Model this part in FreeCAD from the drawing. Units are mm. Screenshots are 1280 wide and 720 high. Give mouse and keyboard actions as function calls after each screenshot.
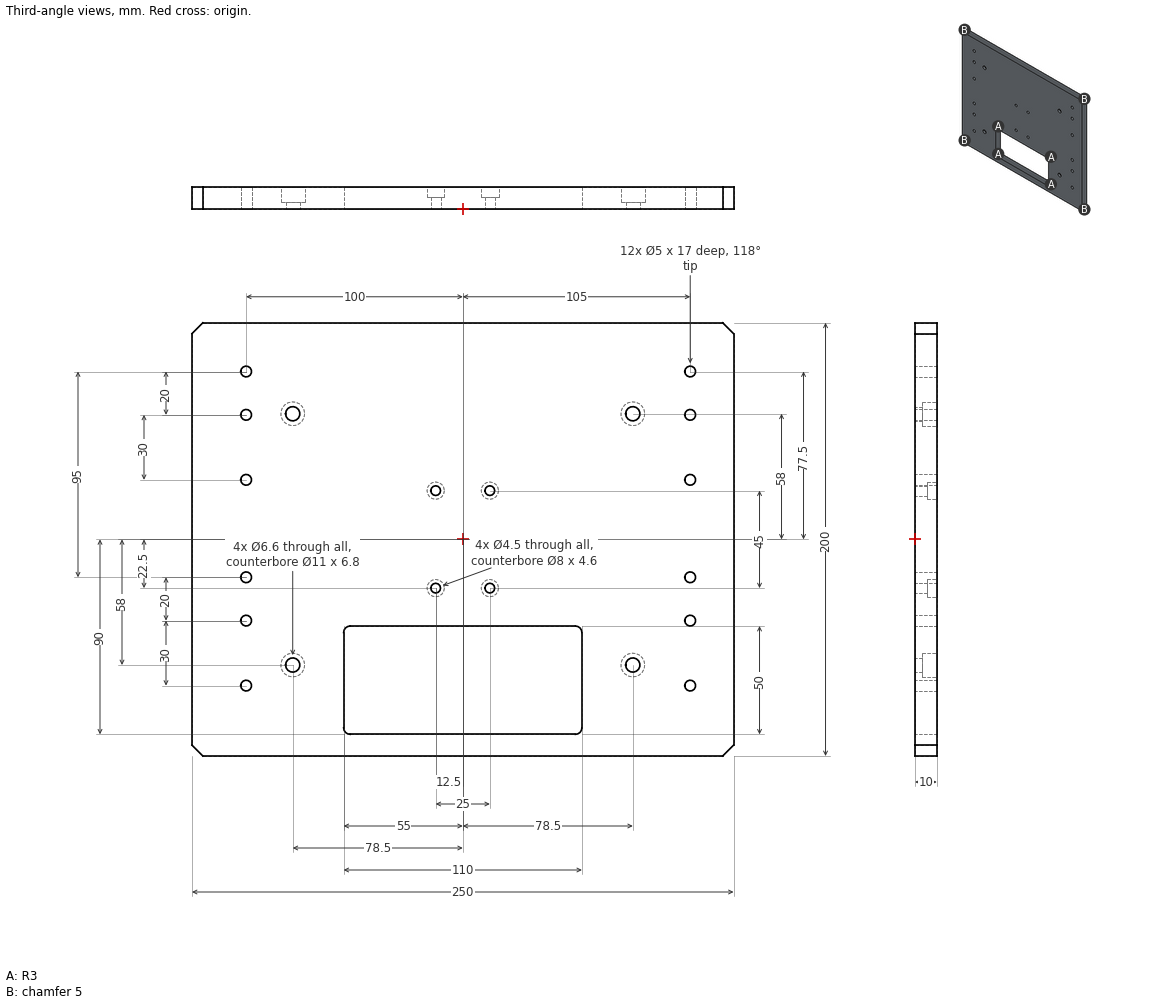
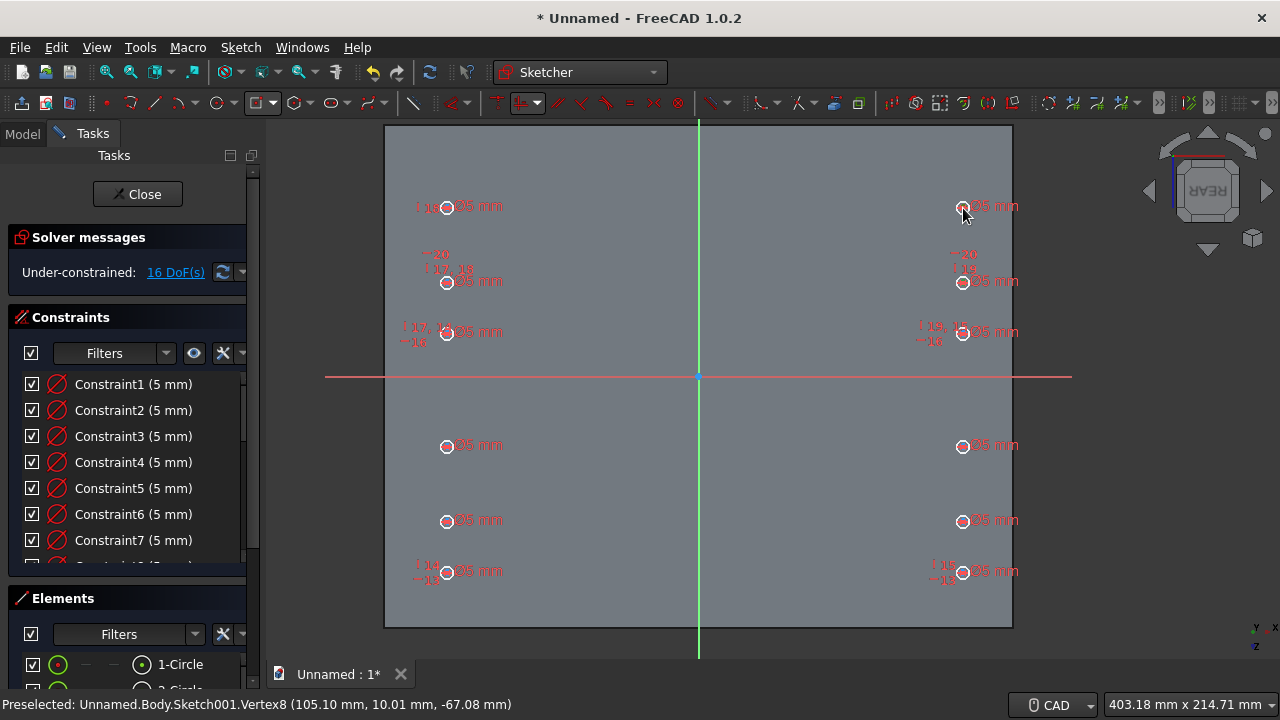
click(540, 104)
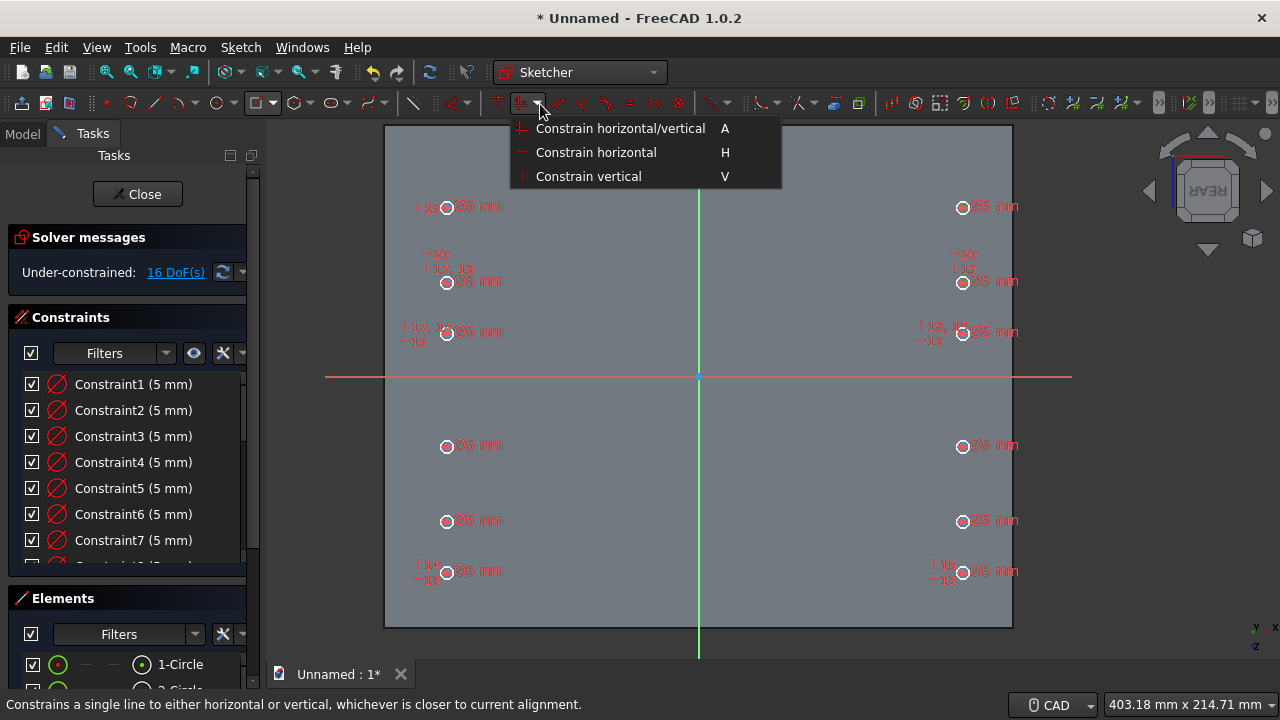
click(646, 176)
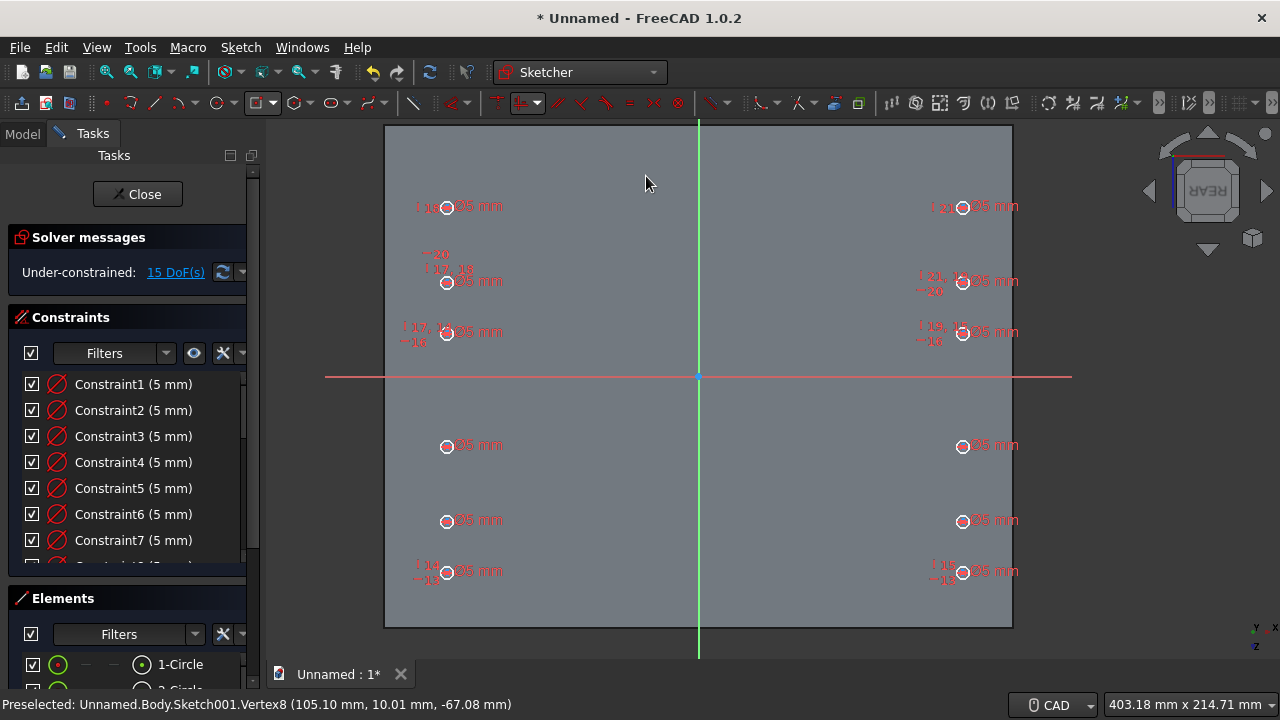
click(447, 208)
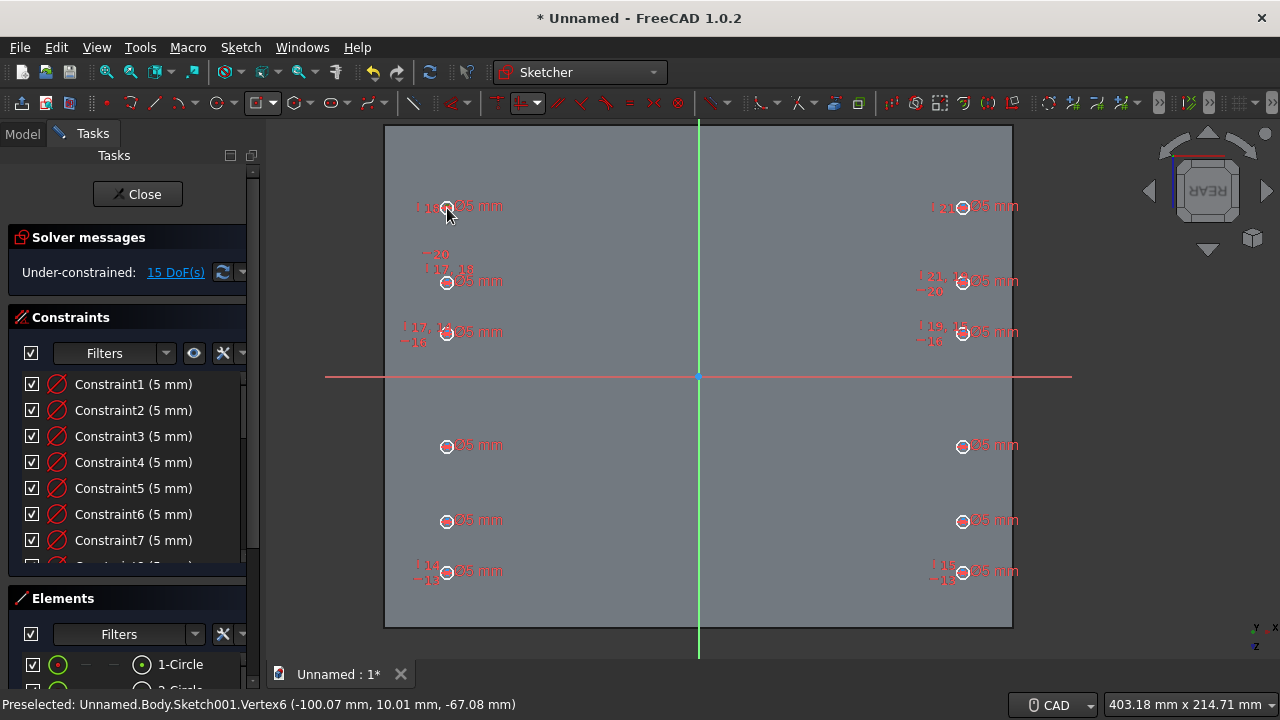
click(963, 208)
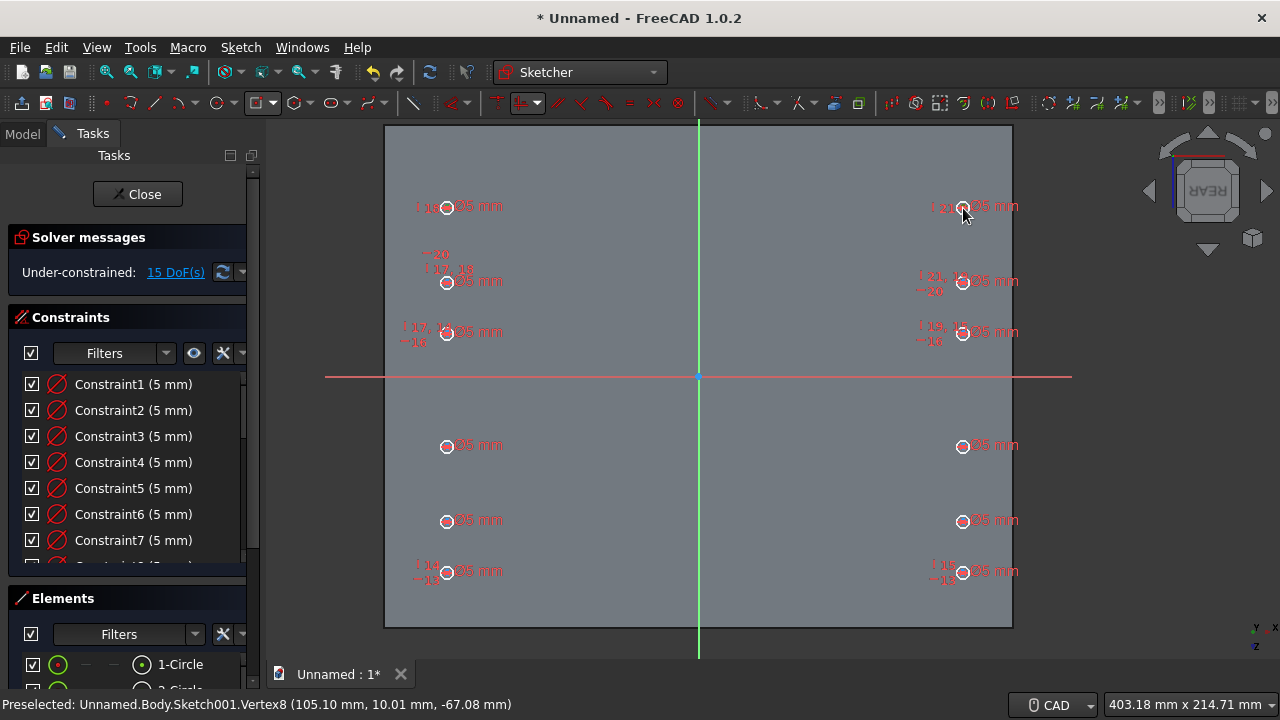
key(h)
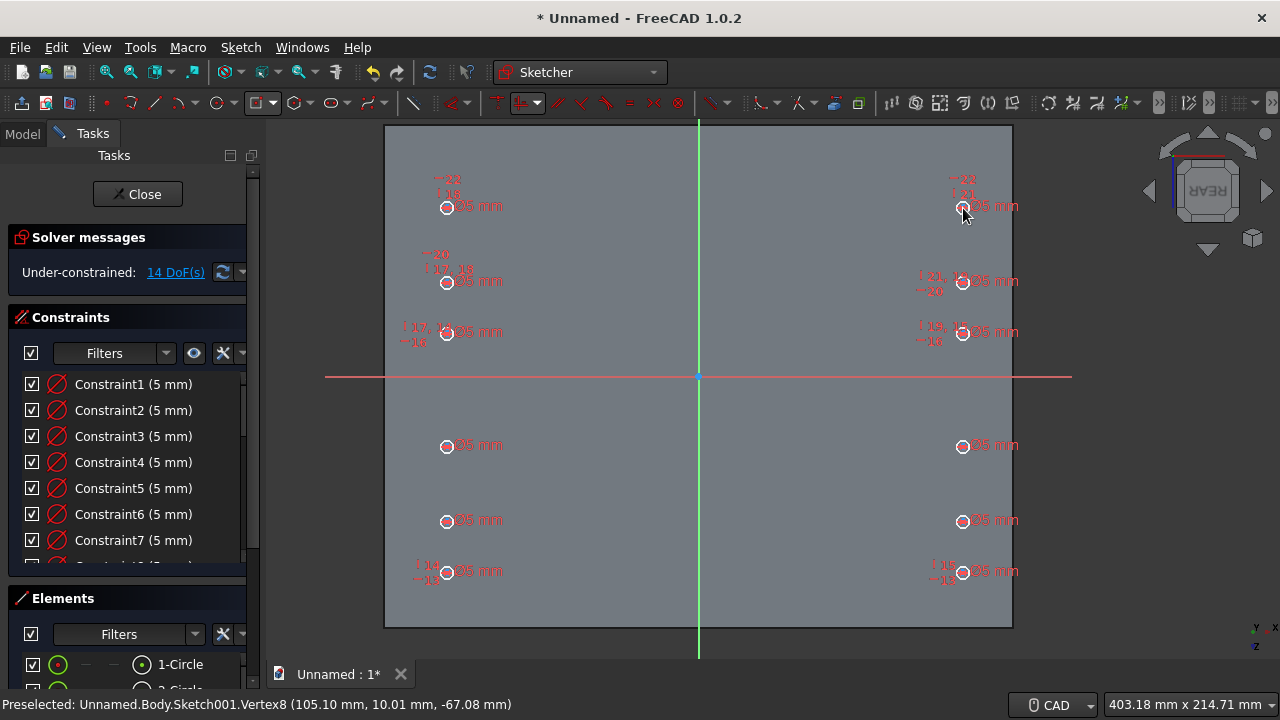
click(447, 573)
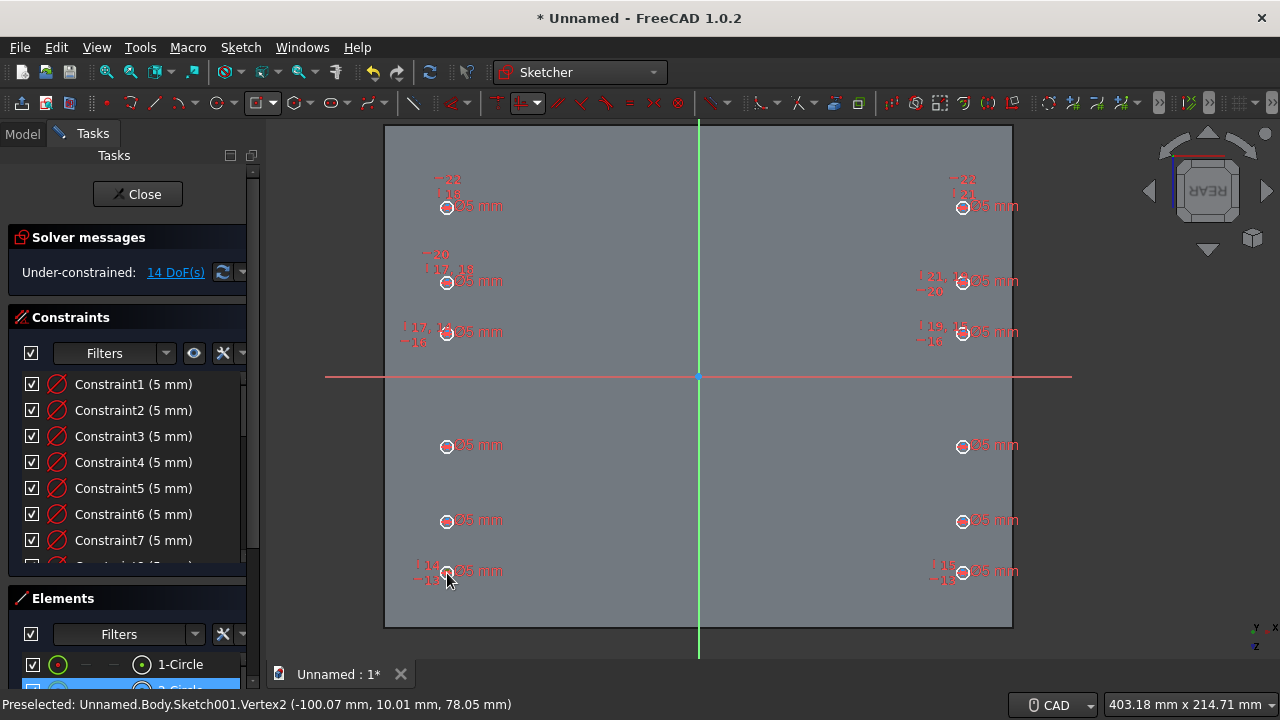
click(447, 522)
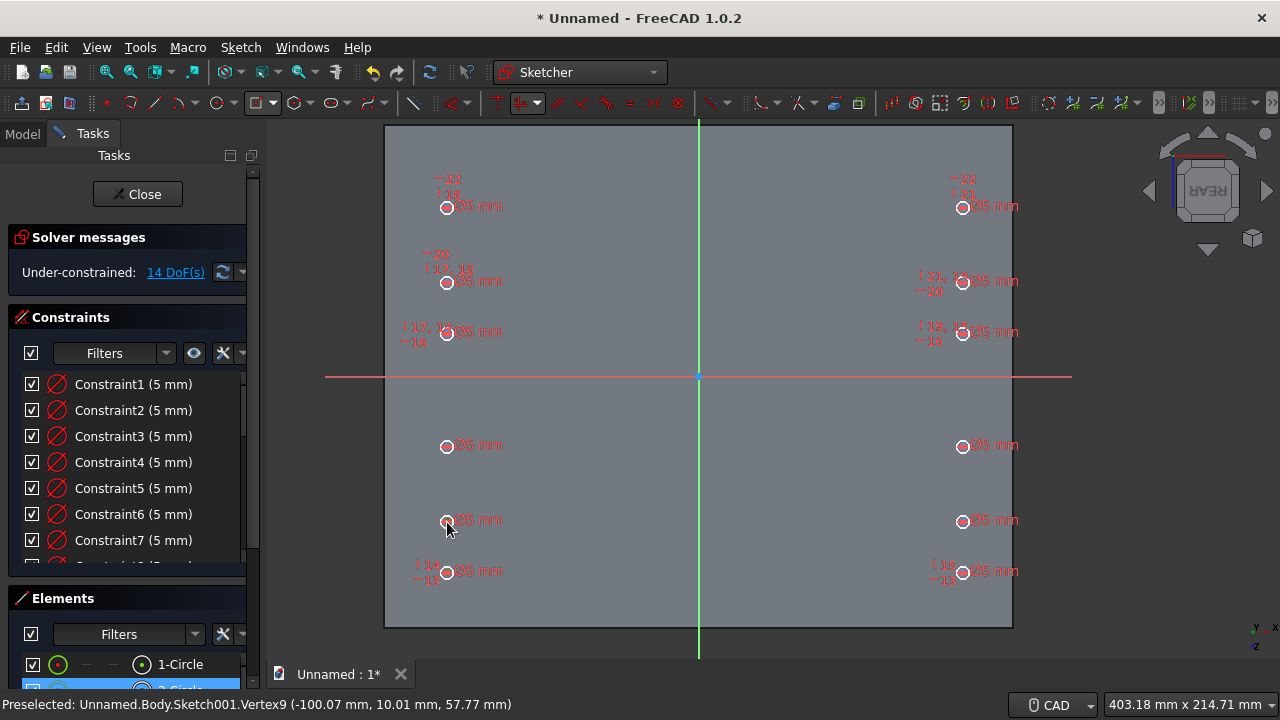
click(540, 104)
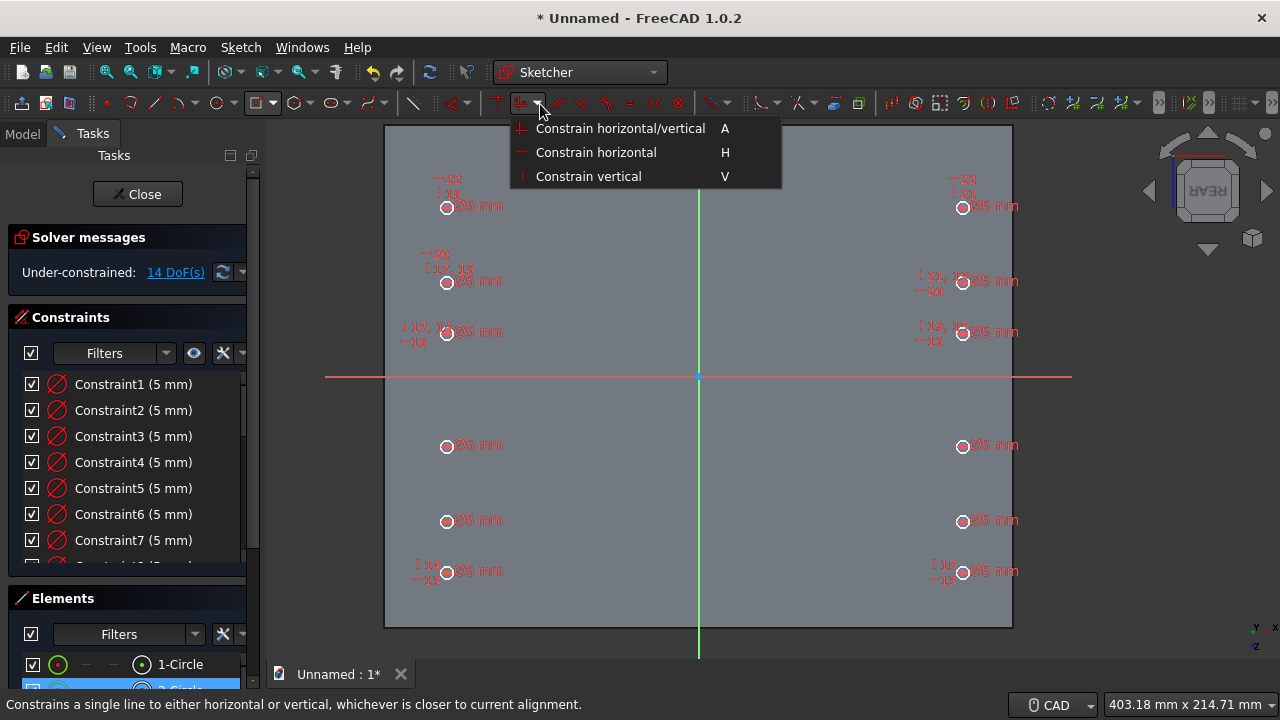
click(646, 176)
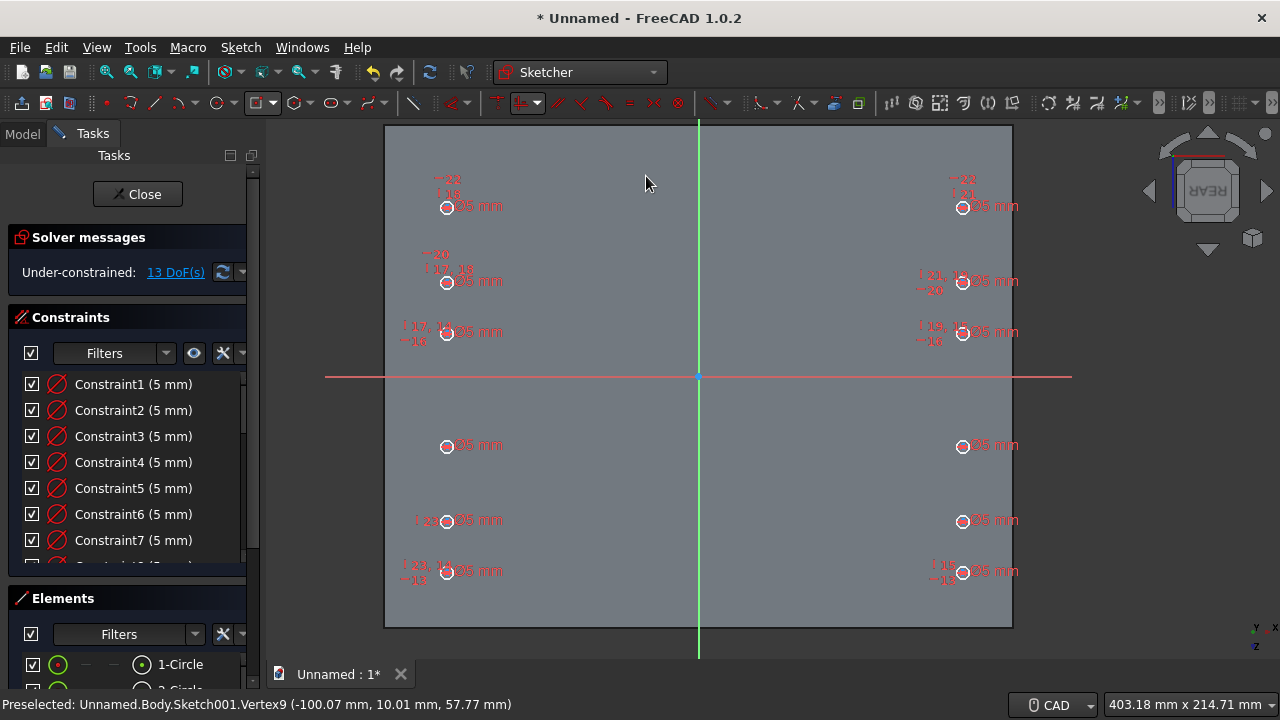
click(447, 522)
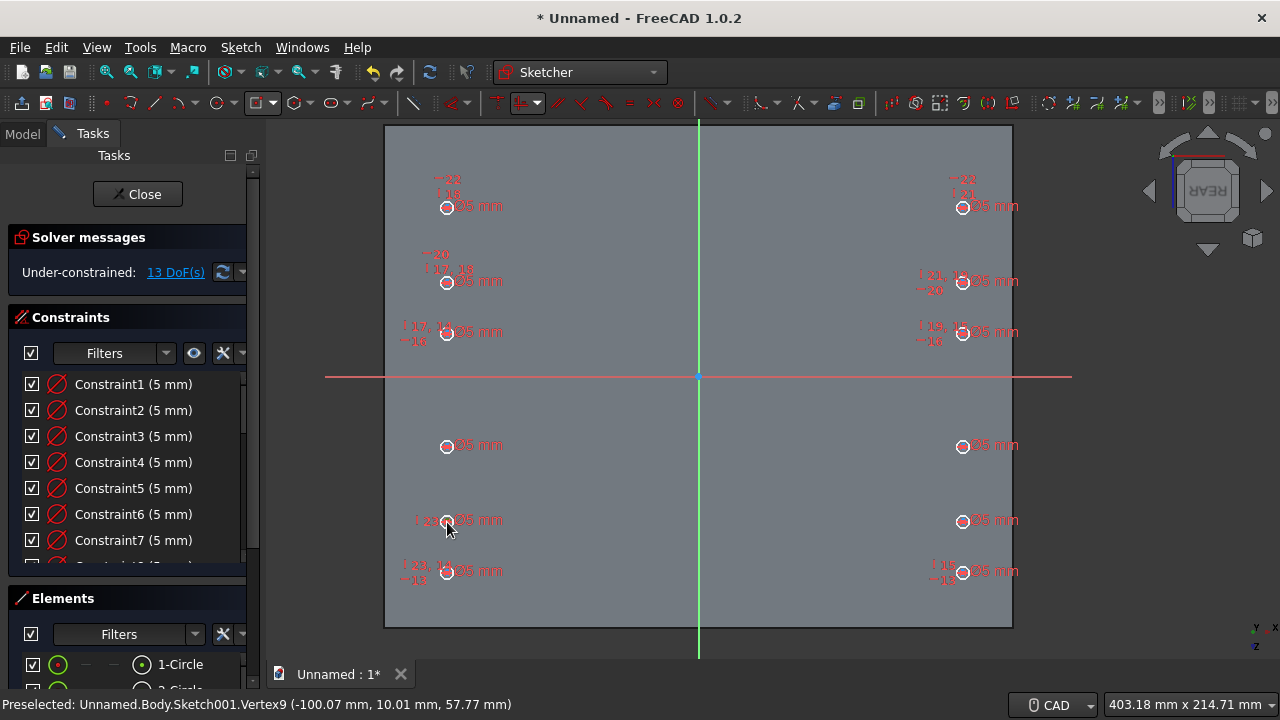
click(447, 447)